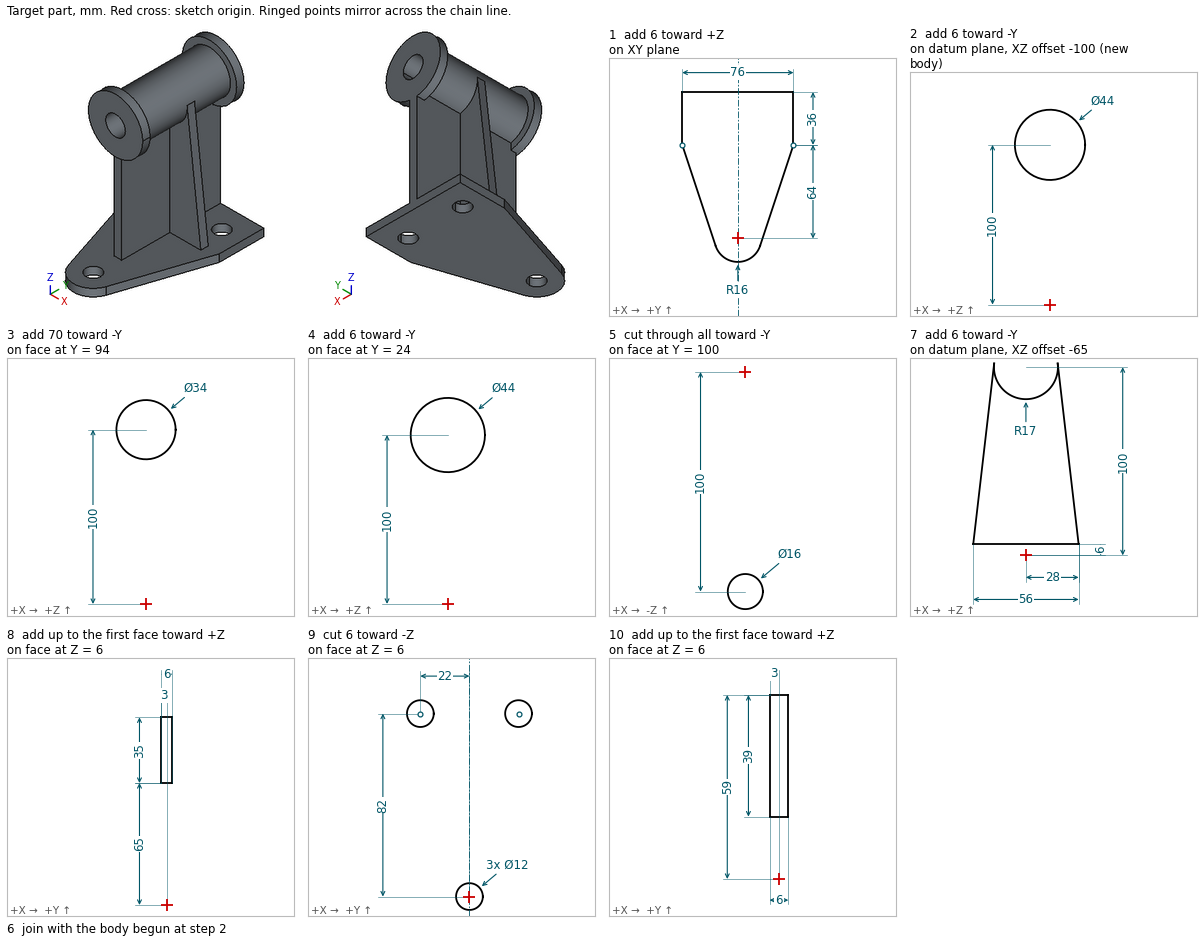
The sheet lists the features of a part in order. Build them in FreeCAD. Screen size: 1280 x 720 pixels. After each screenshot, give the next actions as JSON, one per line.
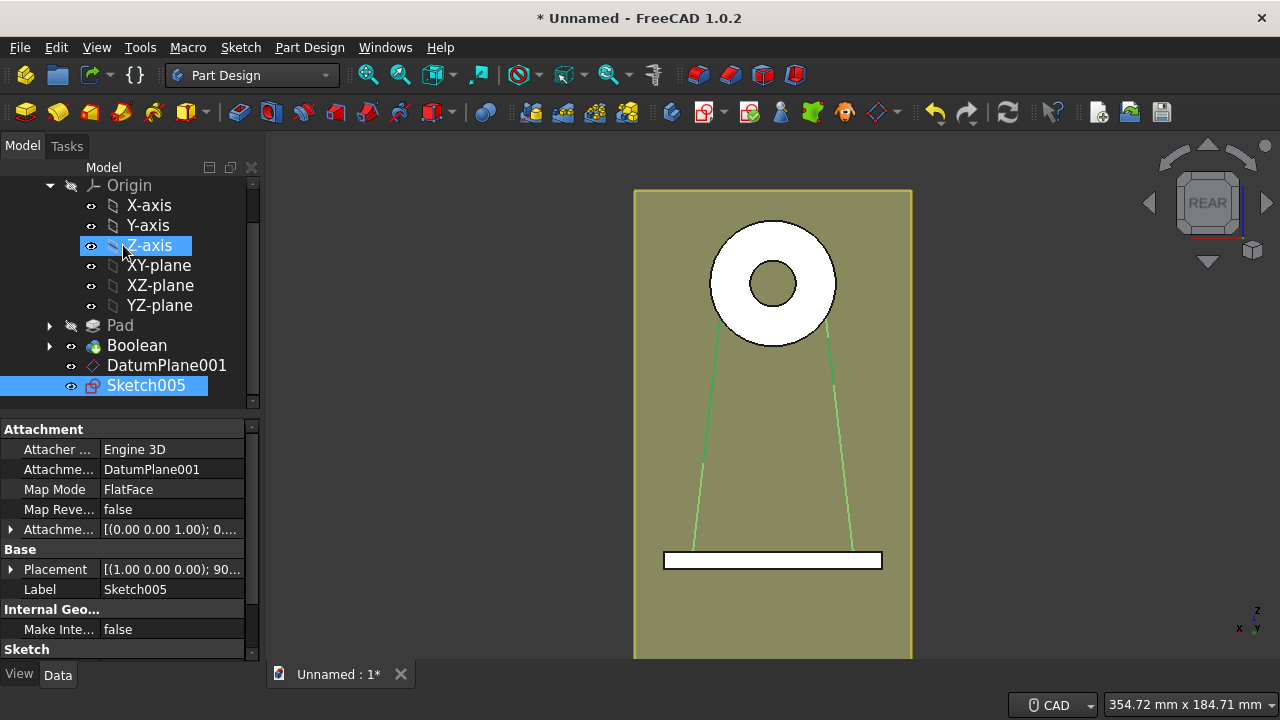
{"action": "left_click", "coordinate": [26, 112]}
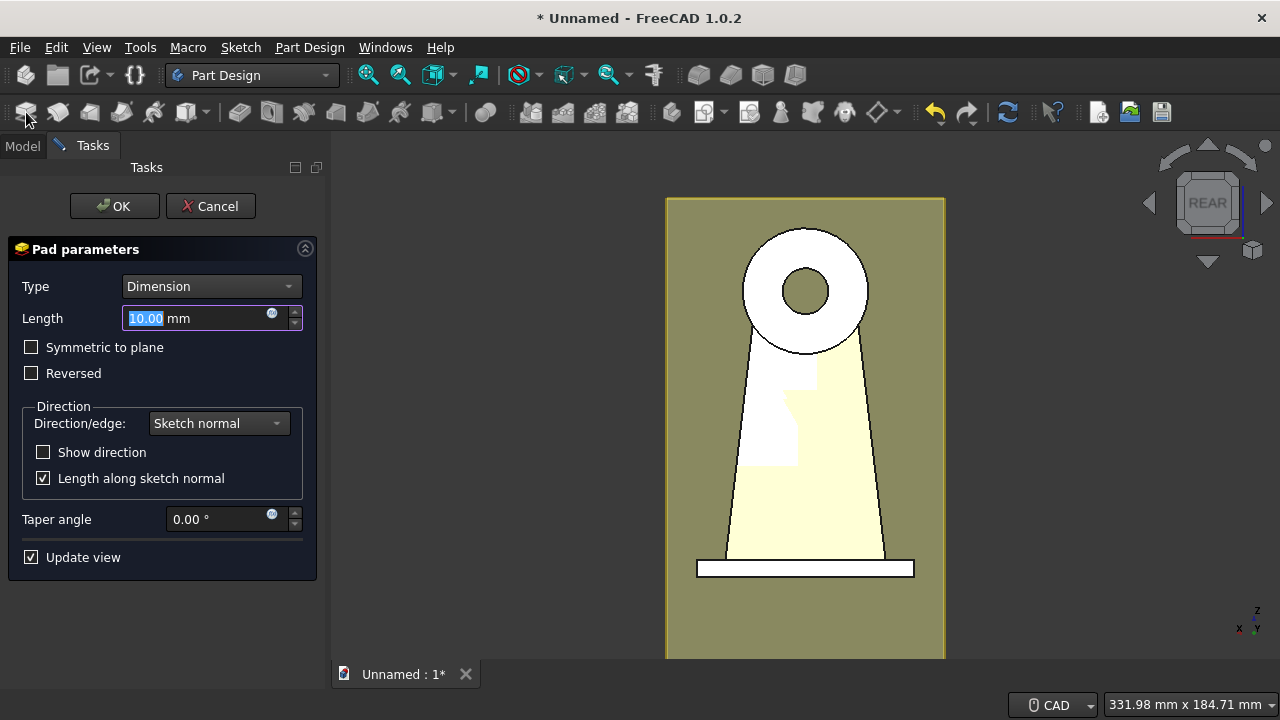
{"action": "type", "text": "6"}
{"action": "key", "text": "Tab"}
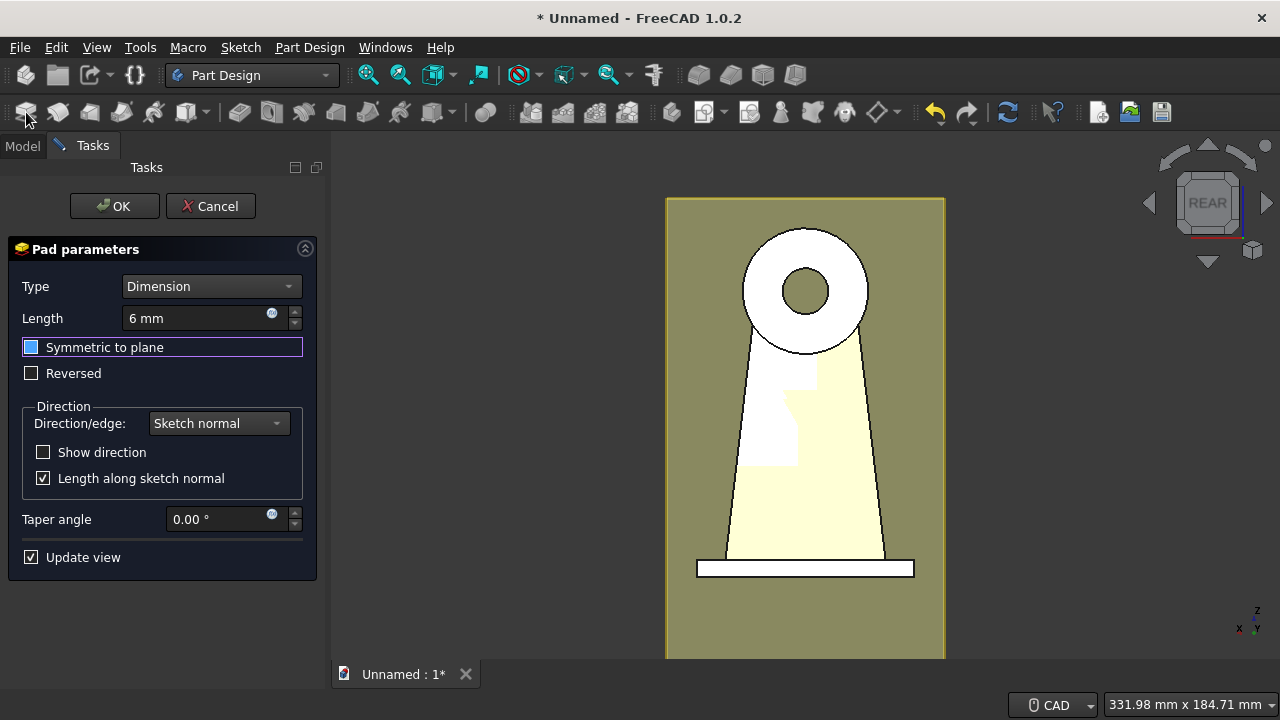
{"action": "left_click", "coordinate": [115, 206]}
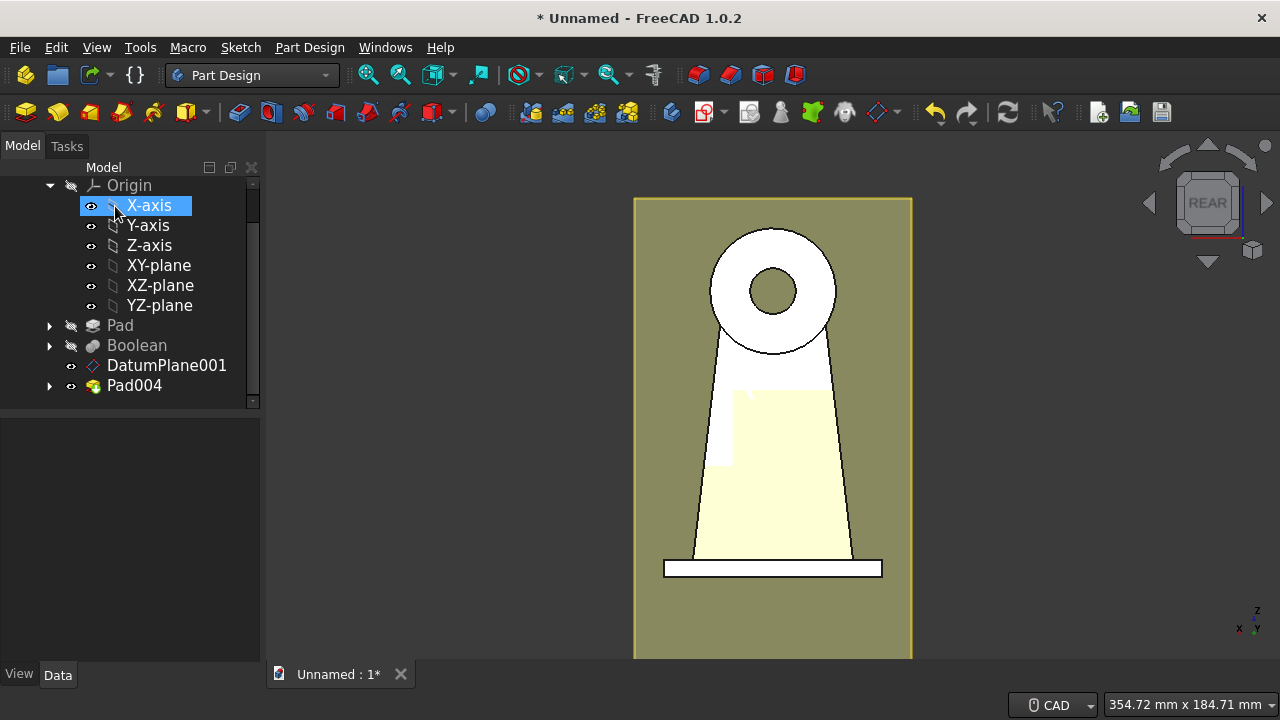
{"action": "left_click", "coordinate": [116, 366]}
{"action": "key", "text": "space"}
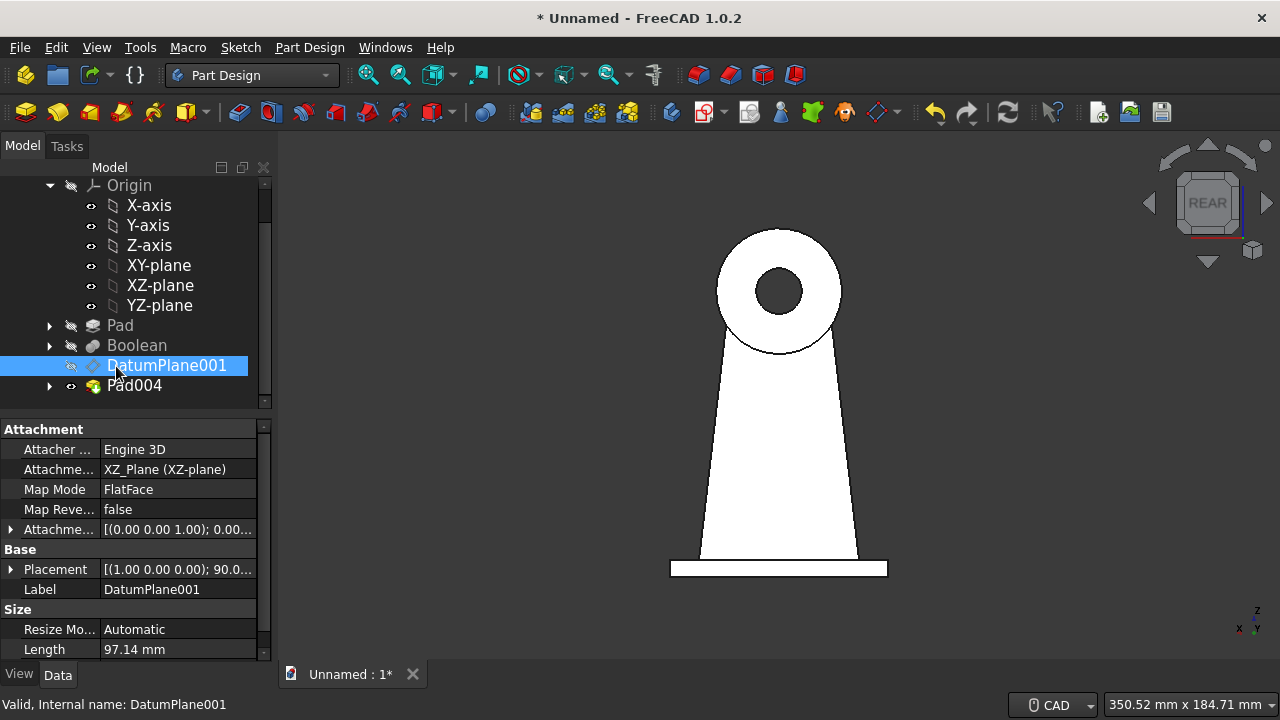
{"action": "key", "text": "0"}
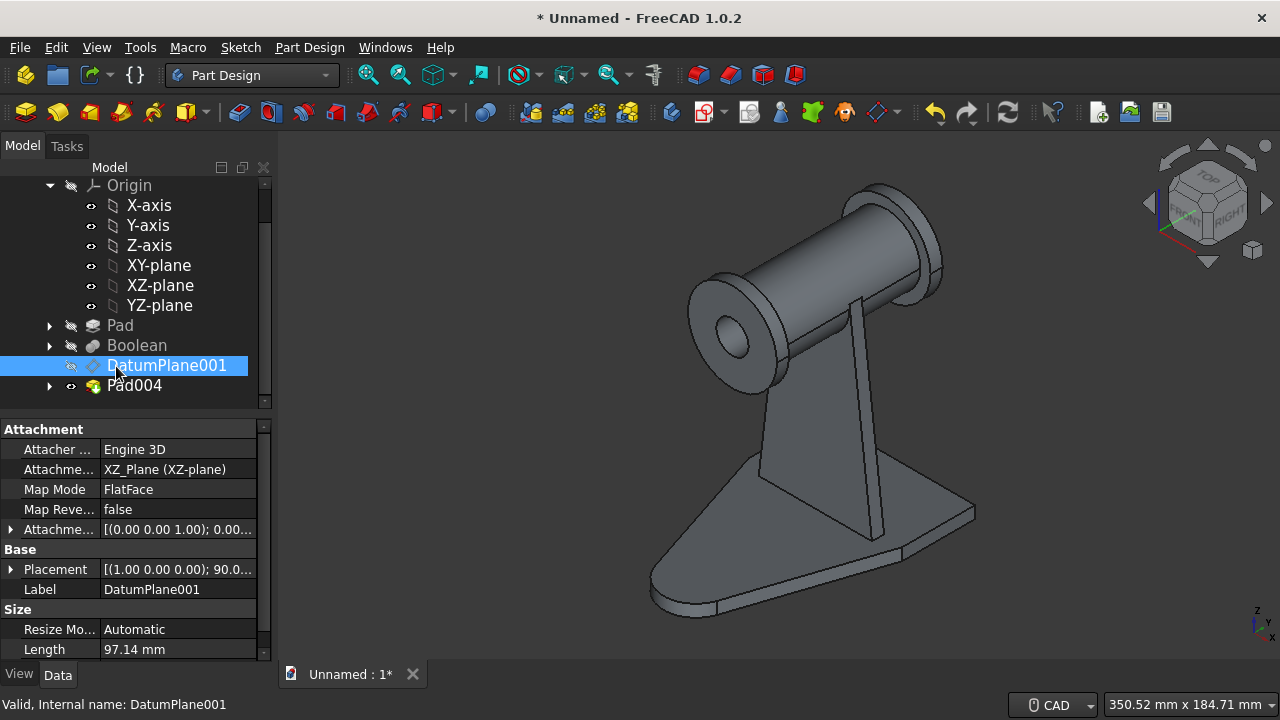
{"action": "left_click", "coordinate": [714, 566]}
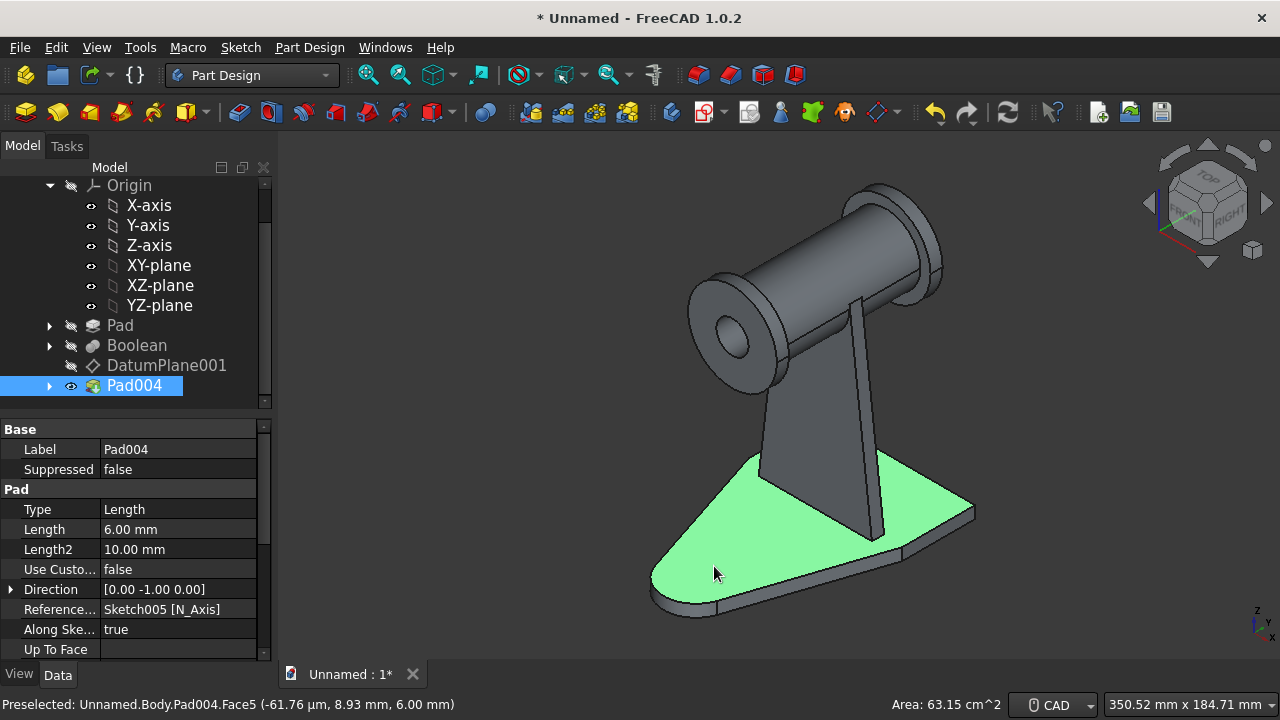
{"action": "left_click", "coordinate": [704, 112]}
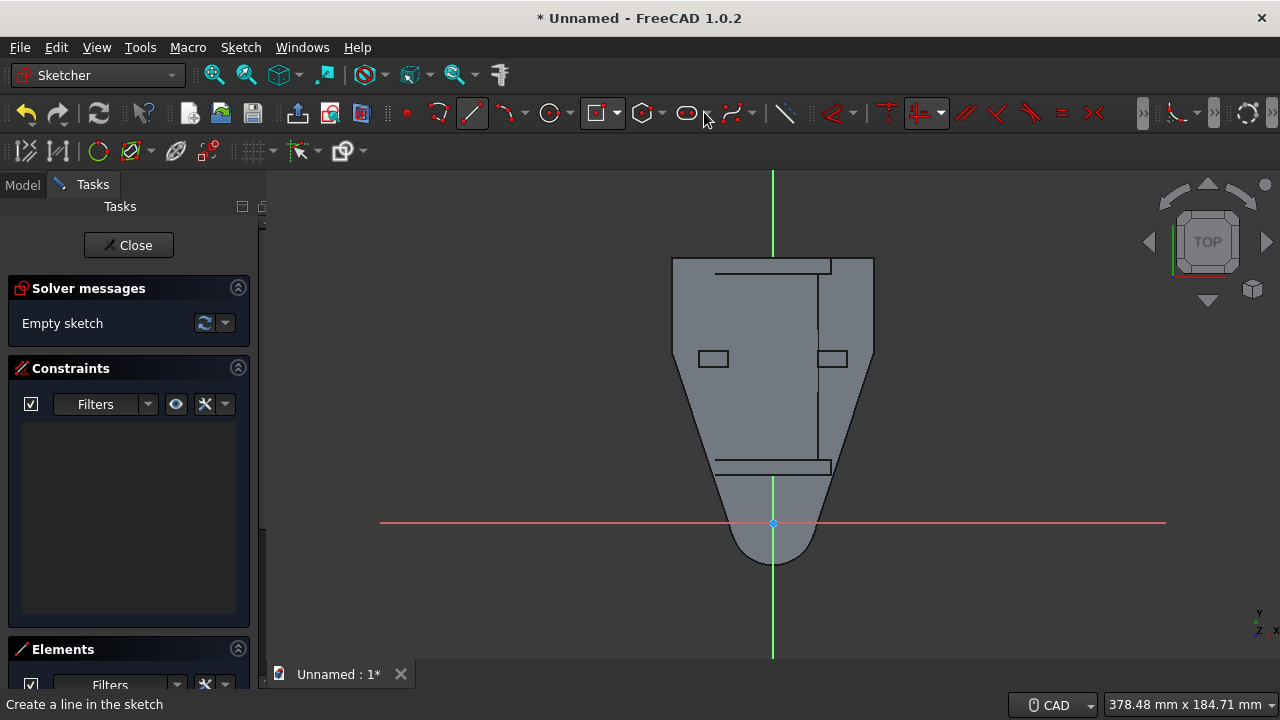
{"action": "scroll", "coordinate": [803, 257], "scroll_direction": "up", "scroll_amount": 6}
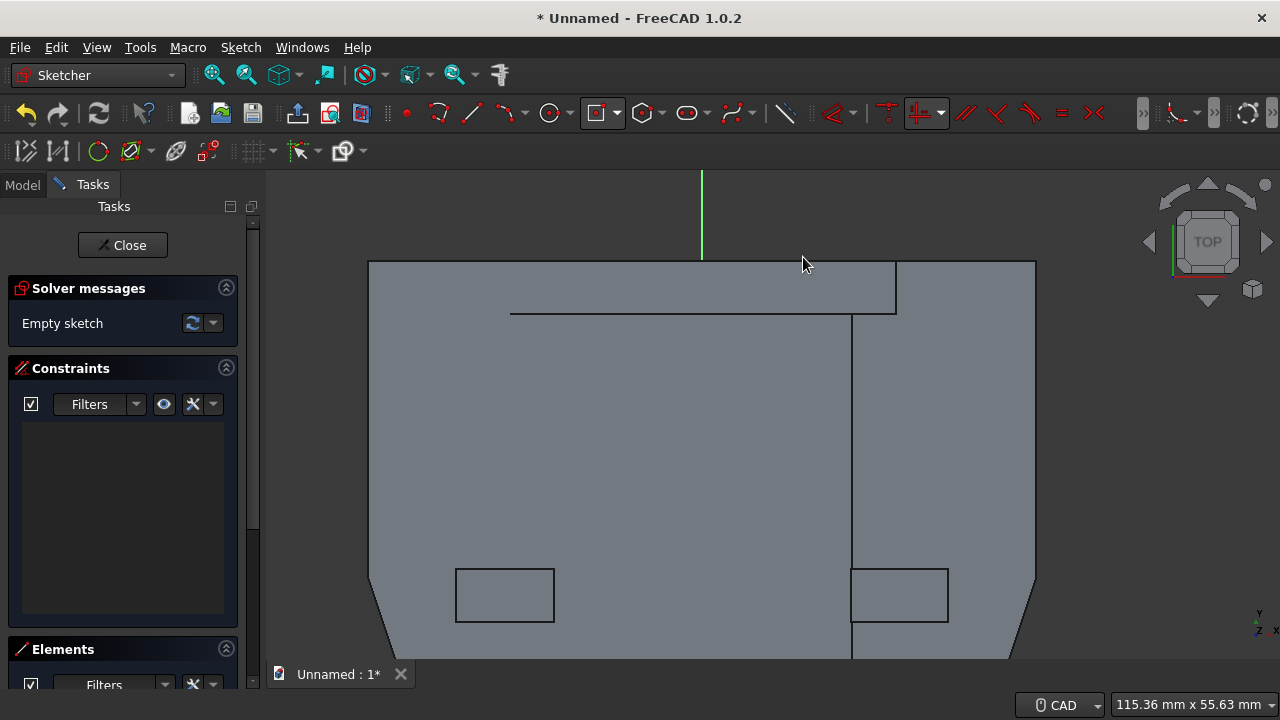
{"action": "key", "text": "g r"}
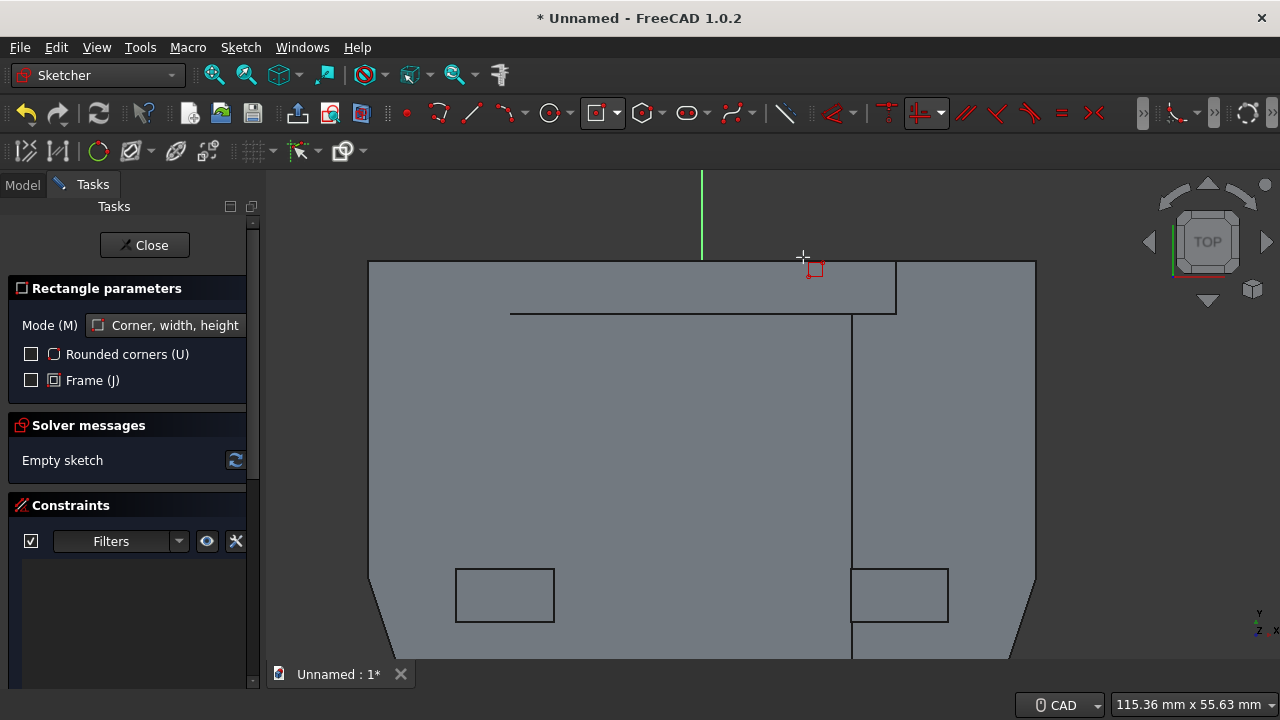
{"action": "left_click", "coordinate": [676, 261]}
{"action": "left_click", "coordinate": [729, 569]}
{"action": "key", "text": "Escape"}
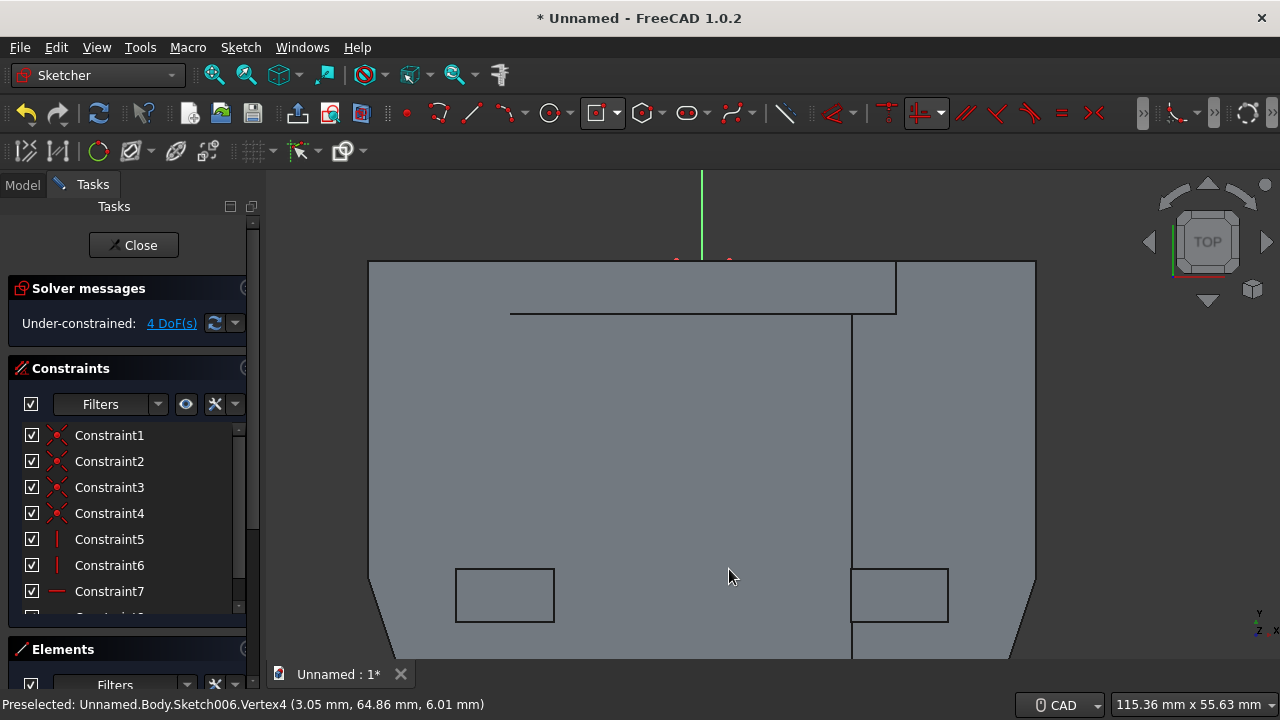
{"action": "key", "text": "d"}